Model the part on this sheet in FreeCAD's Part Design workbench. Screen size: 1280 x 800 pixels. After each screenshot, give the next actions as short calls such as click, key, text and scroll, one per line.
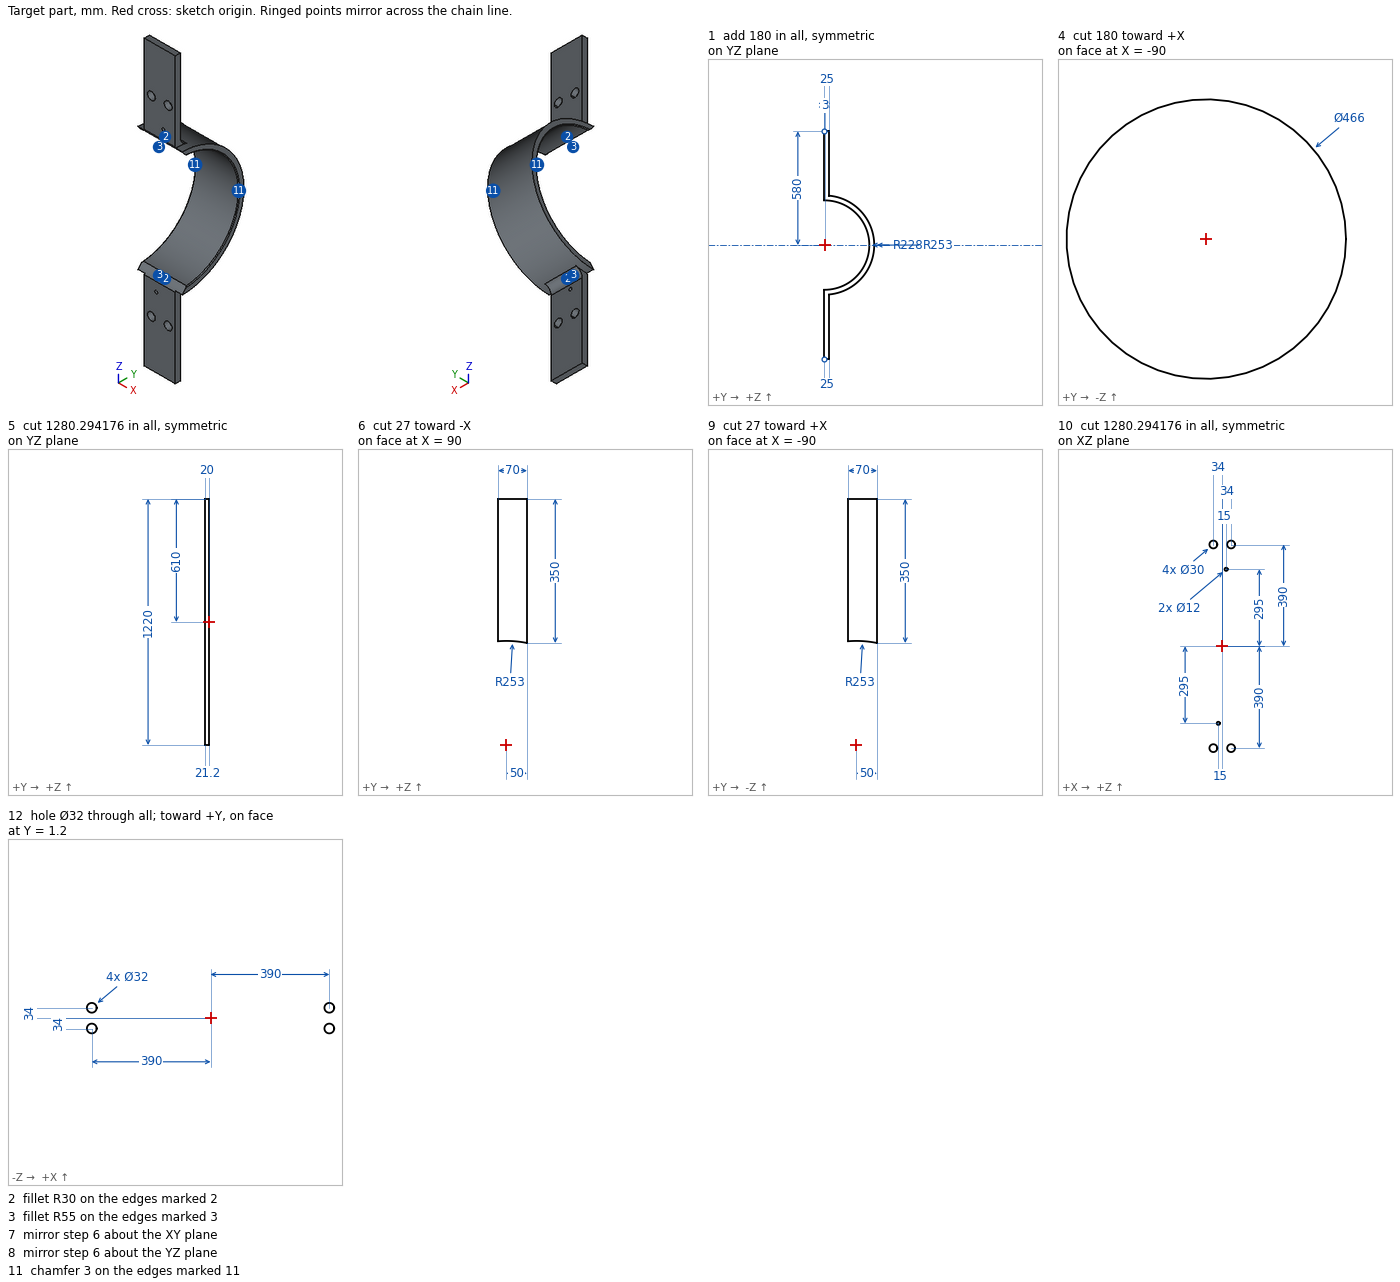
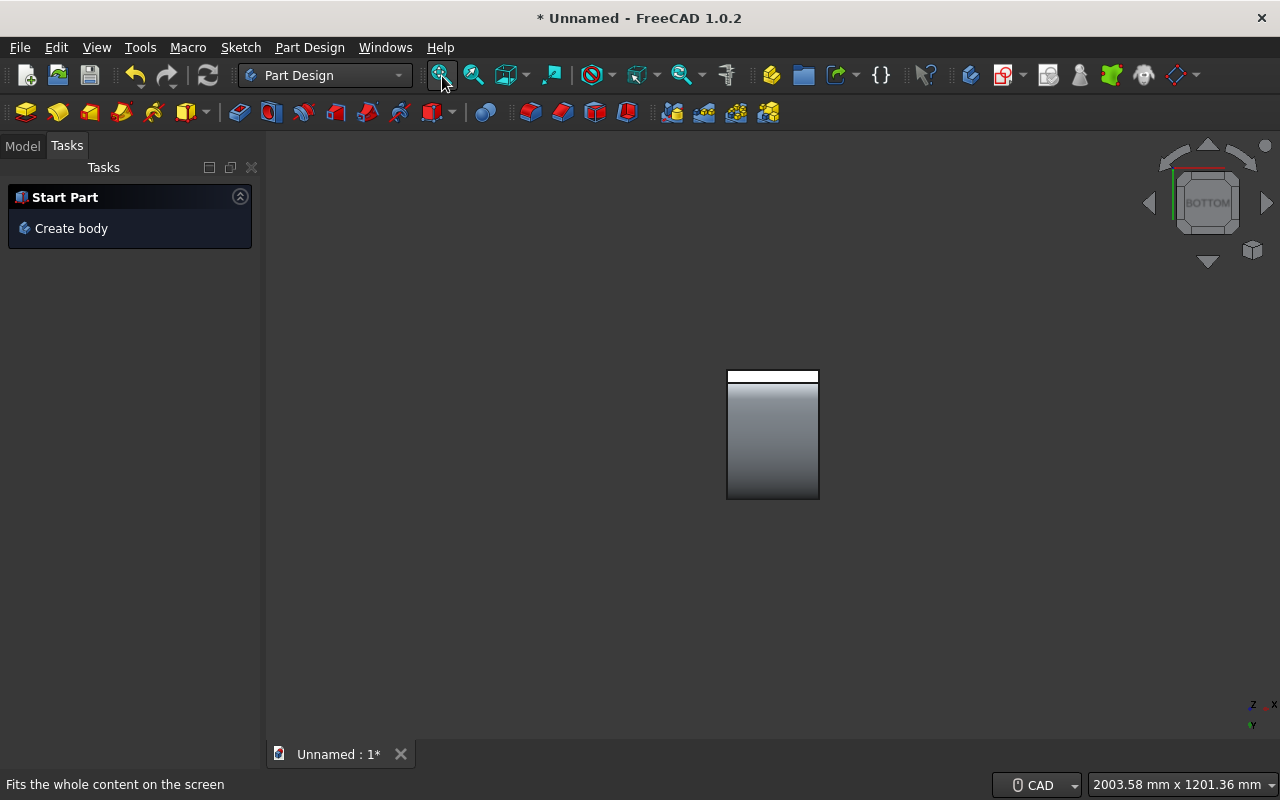
key(4)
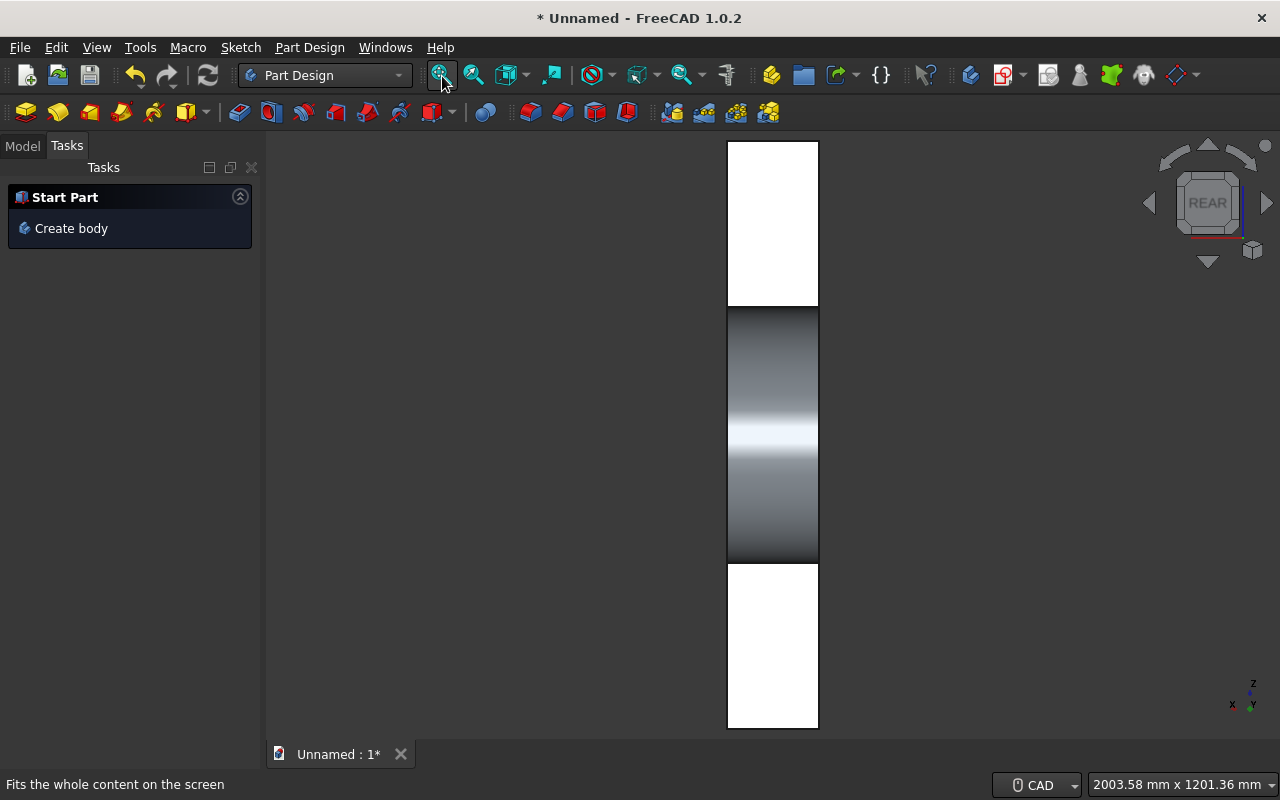
key(6)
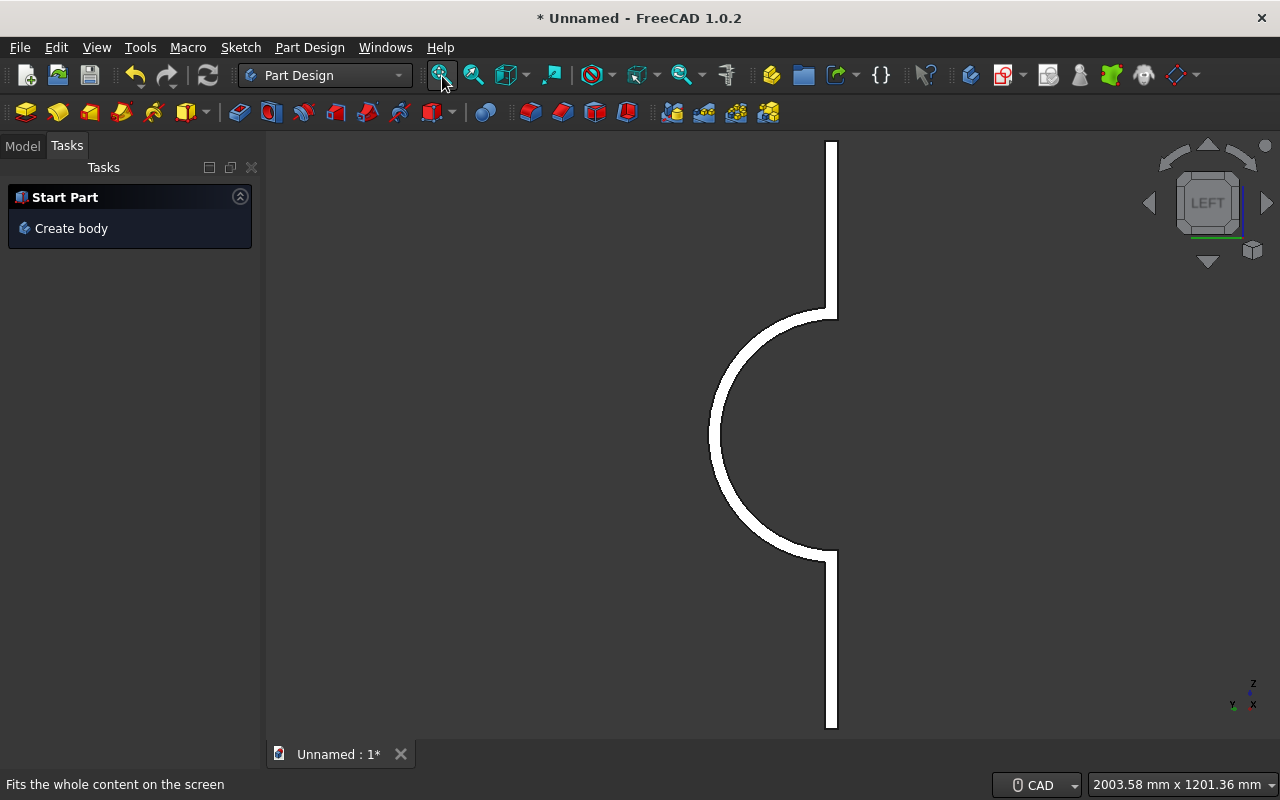
key(v)
key(3)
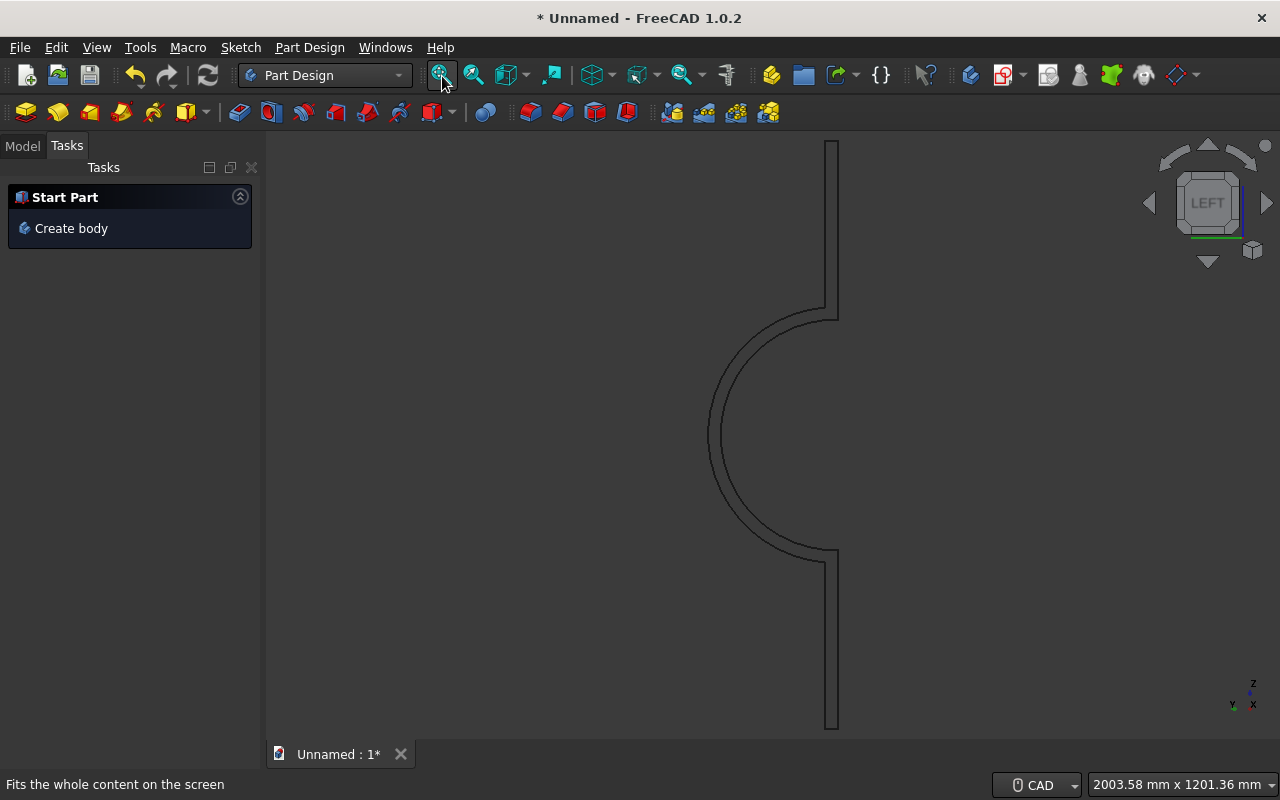
key(0)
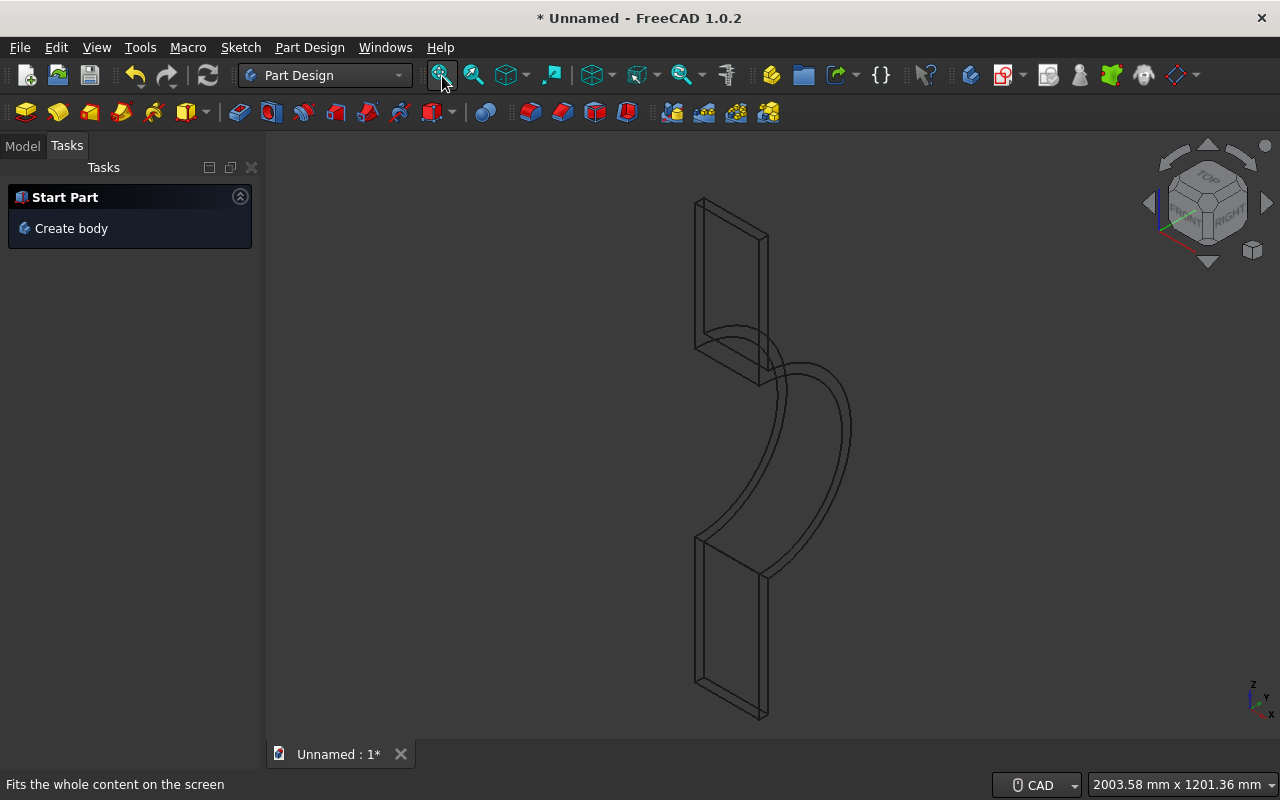
click(736, 351)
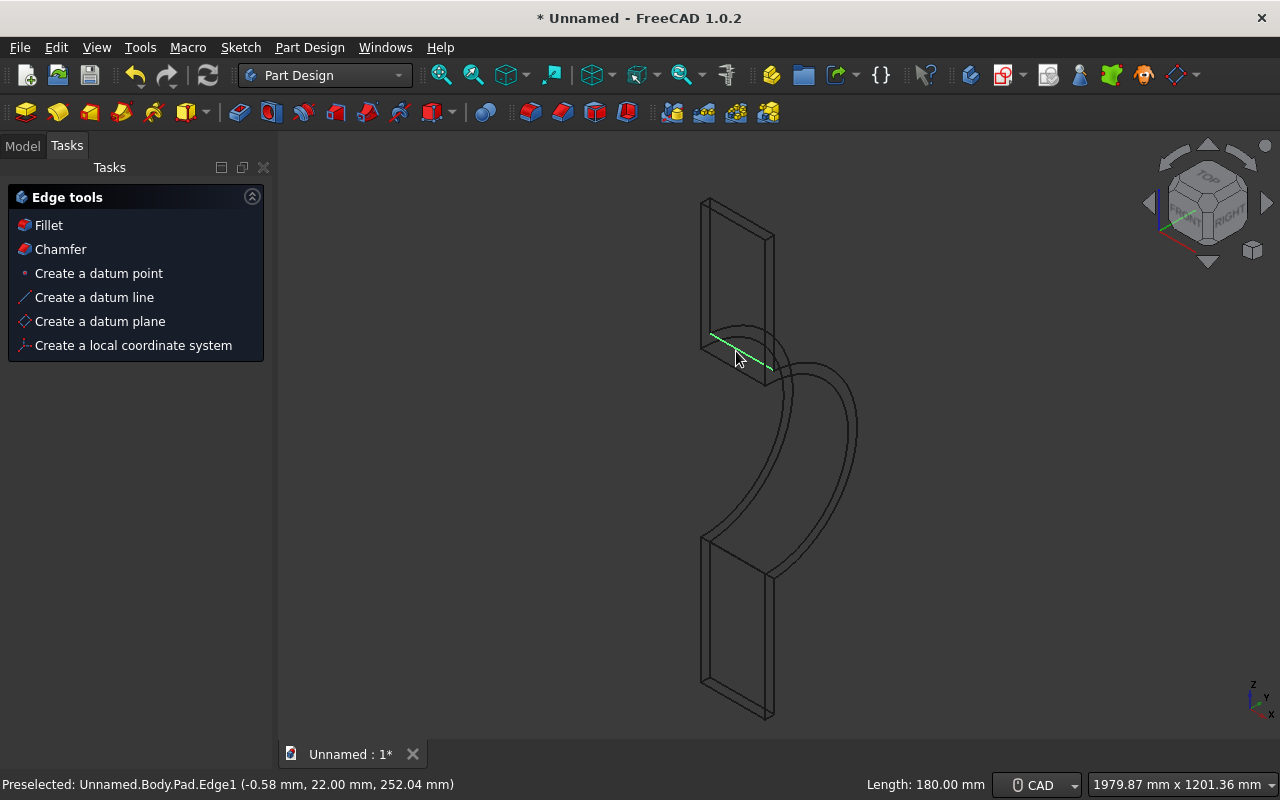
scroll(742, 559, up, 6)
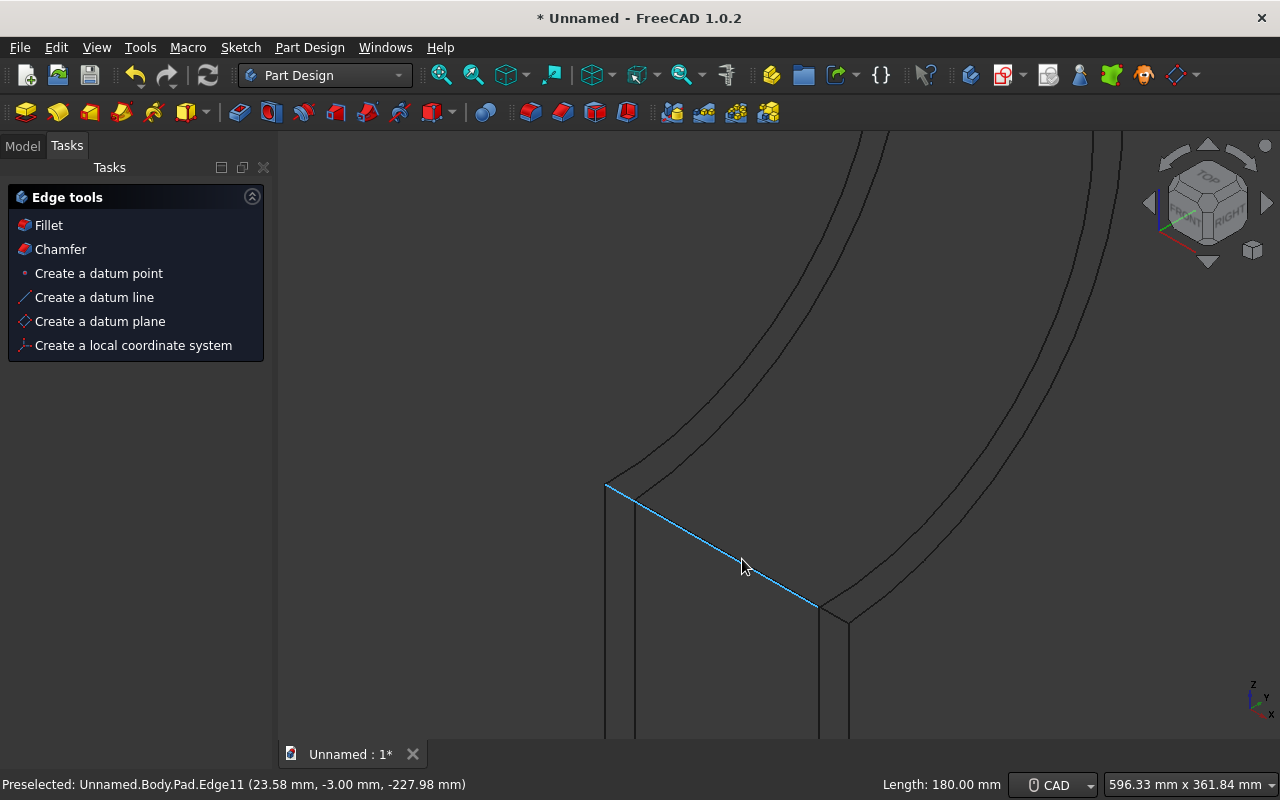
click(442, 76)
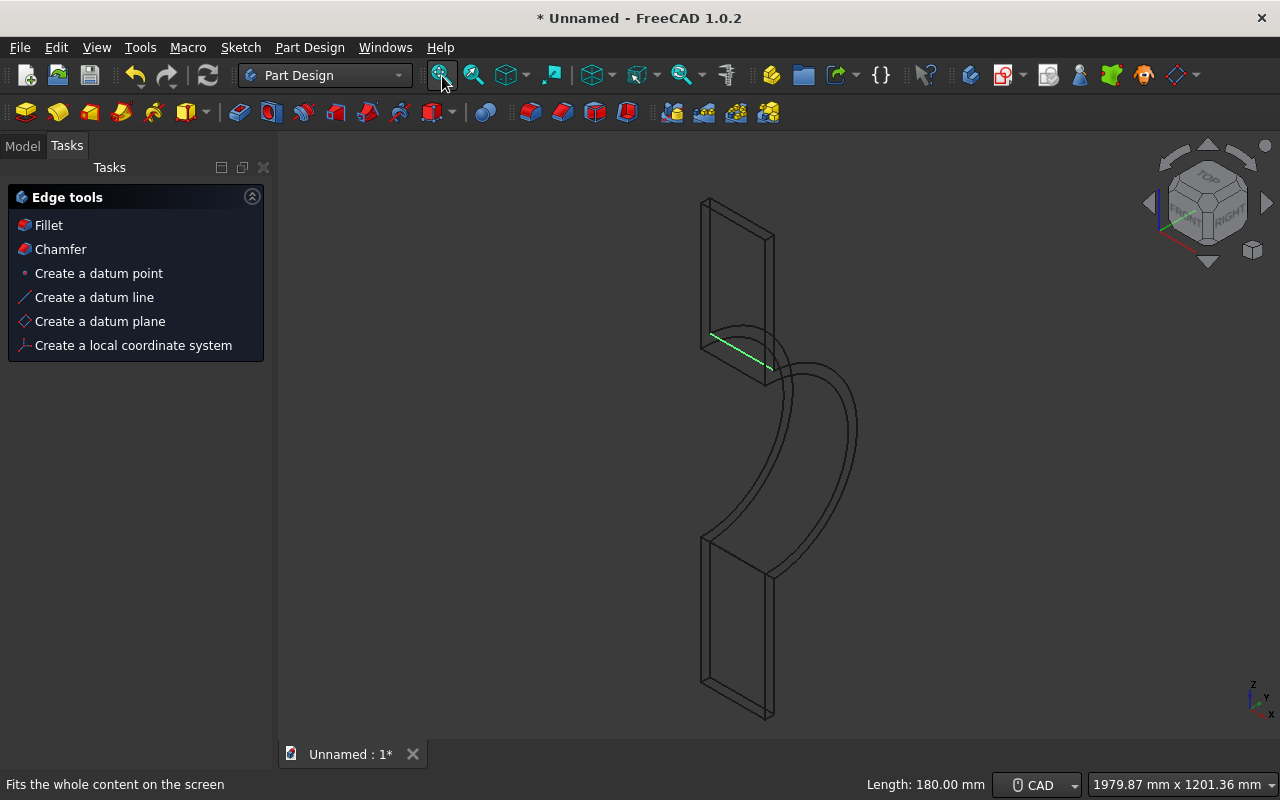
key(2)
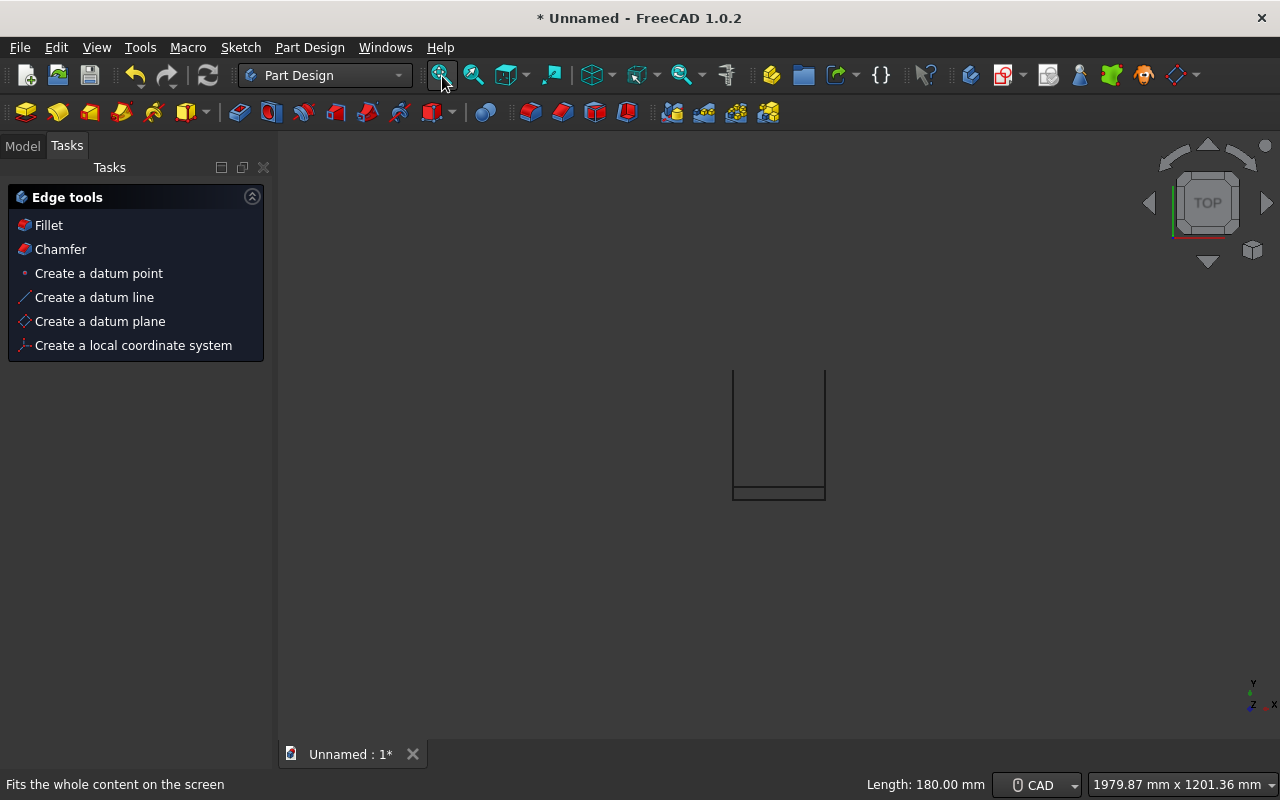
click(442, 76)